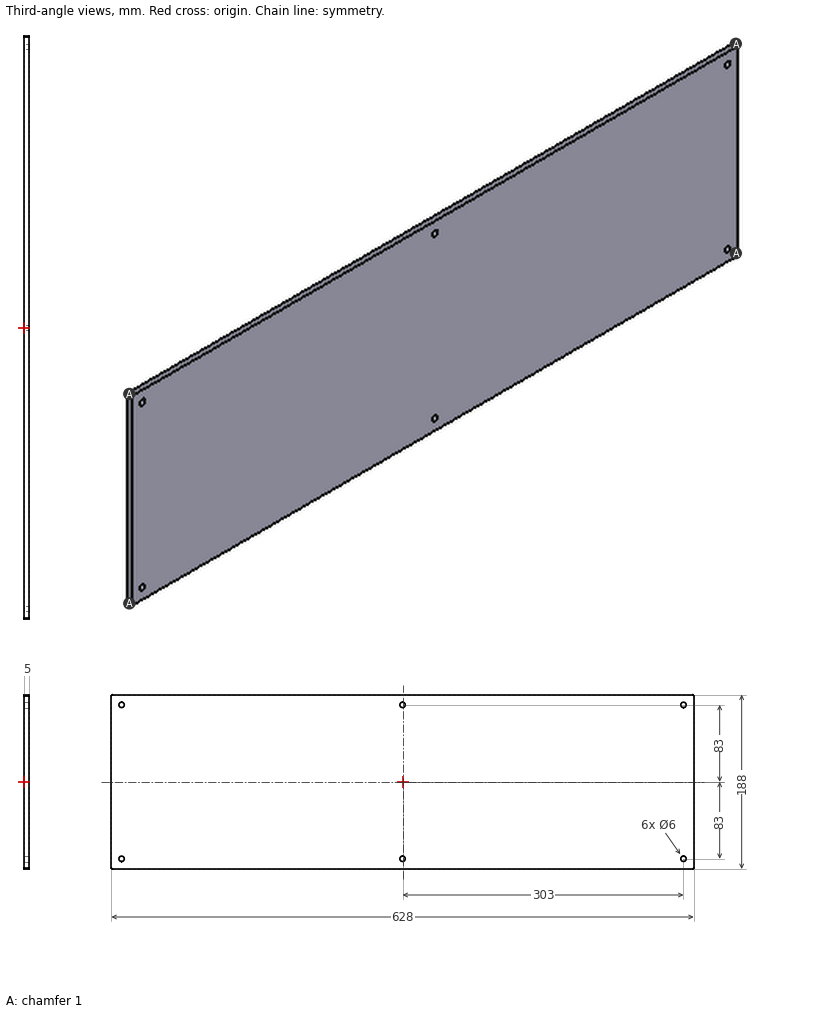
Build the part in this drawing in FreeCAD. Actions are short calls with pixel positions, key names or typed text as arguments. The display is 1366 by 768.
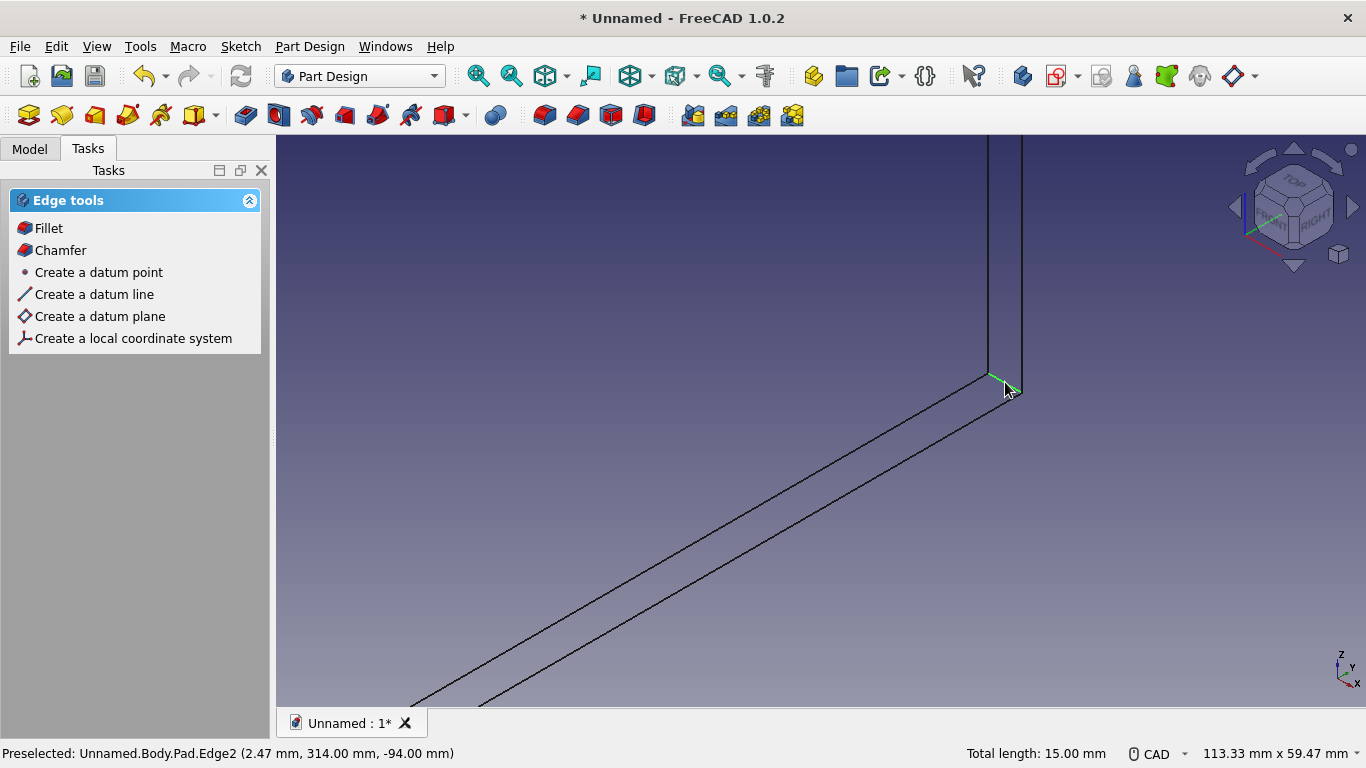
key(v)
key(f)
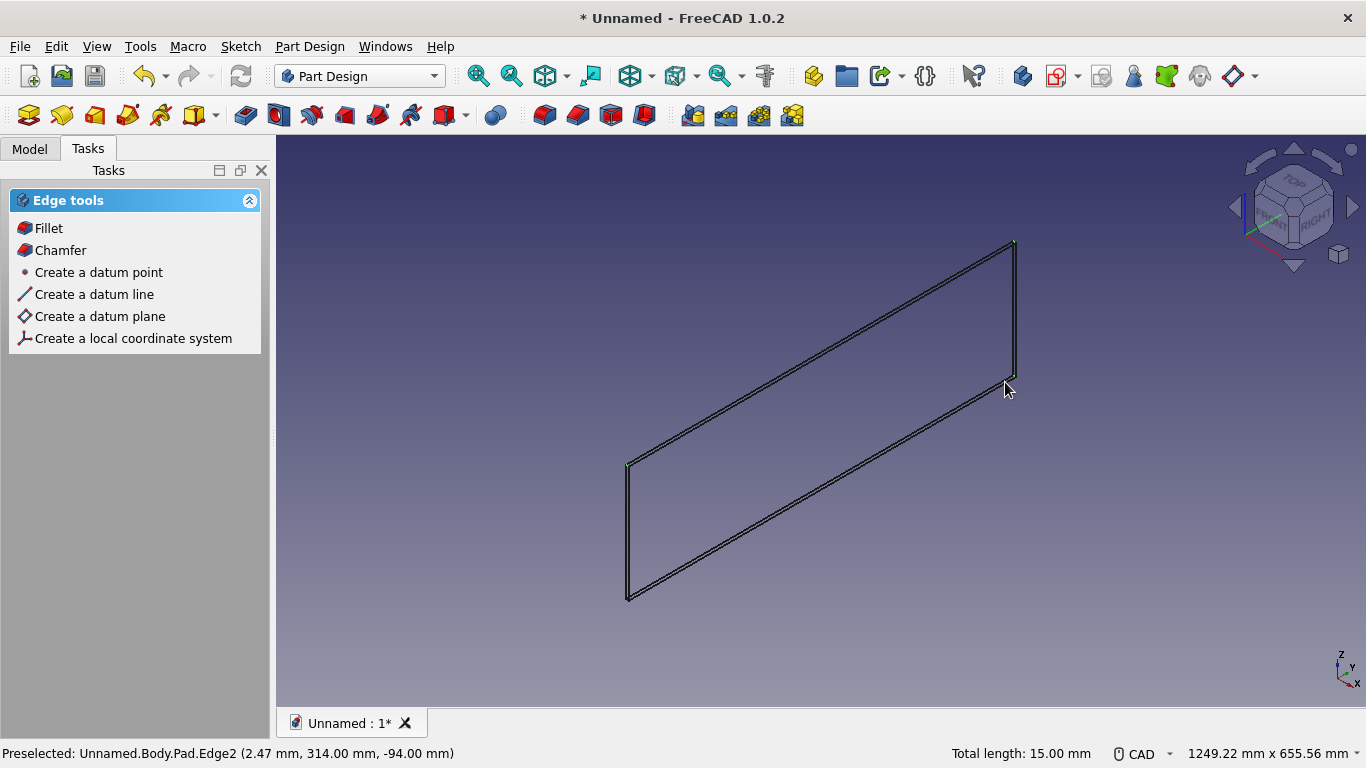
key(2)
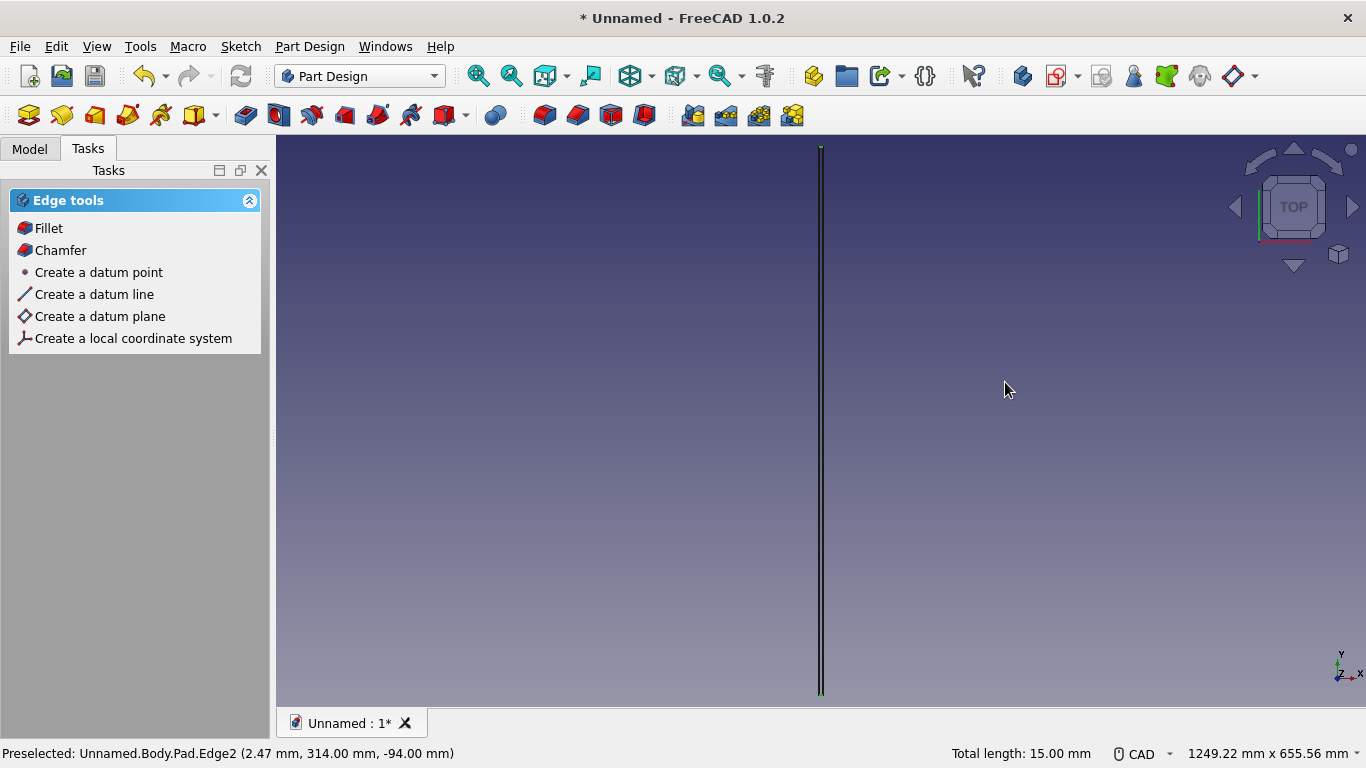
key(1)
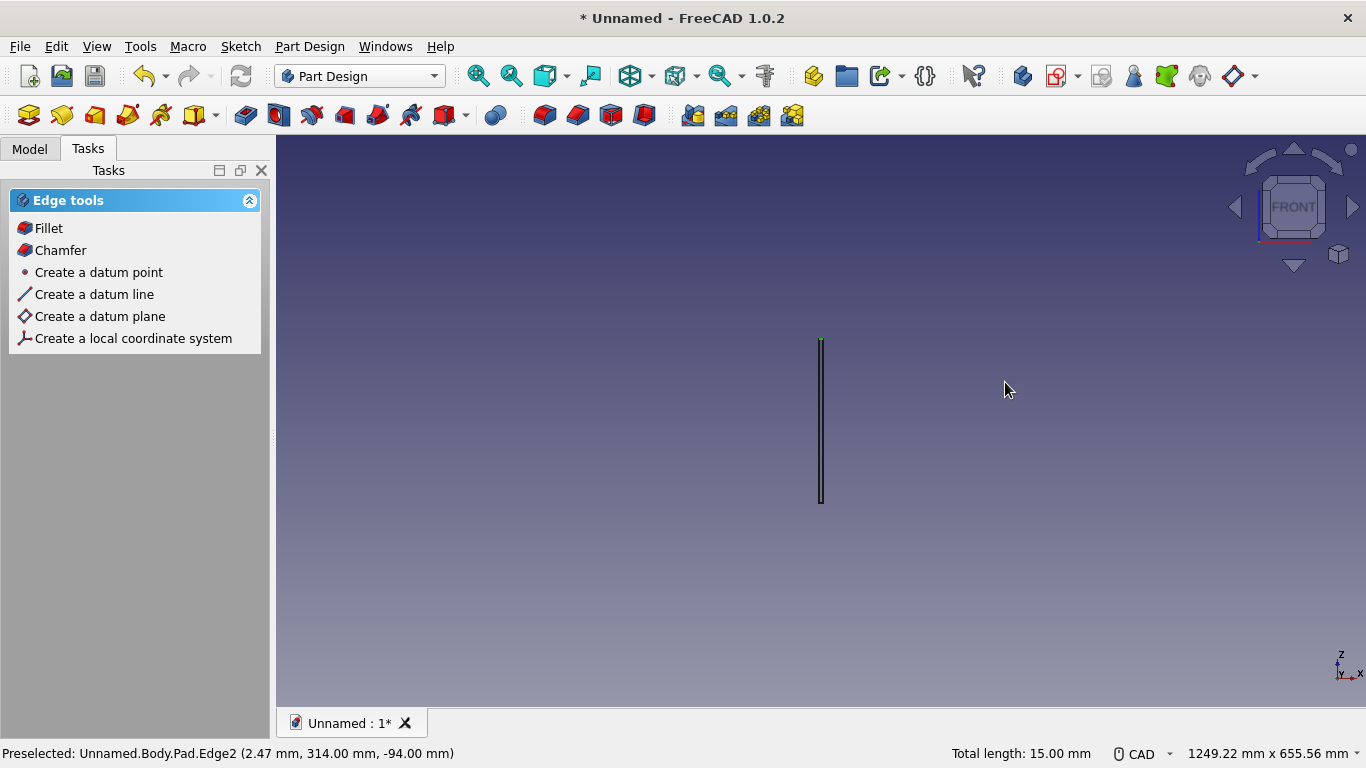
key(v)
key(f)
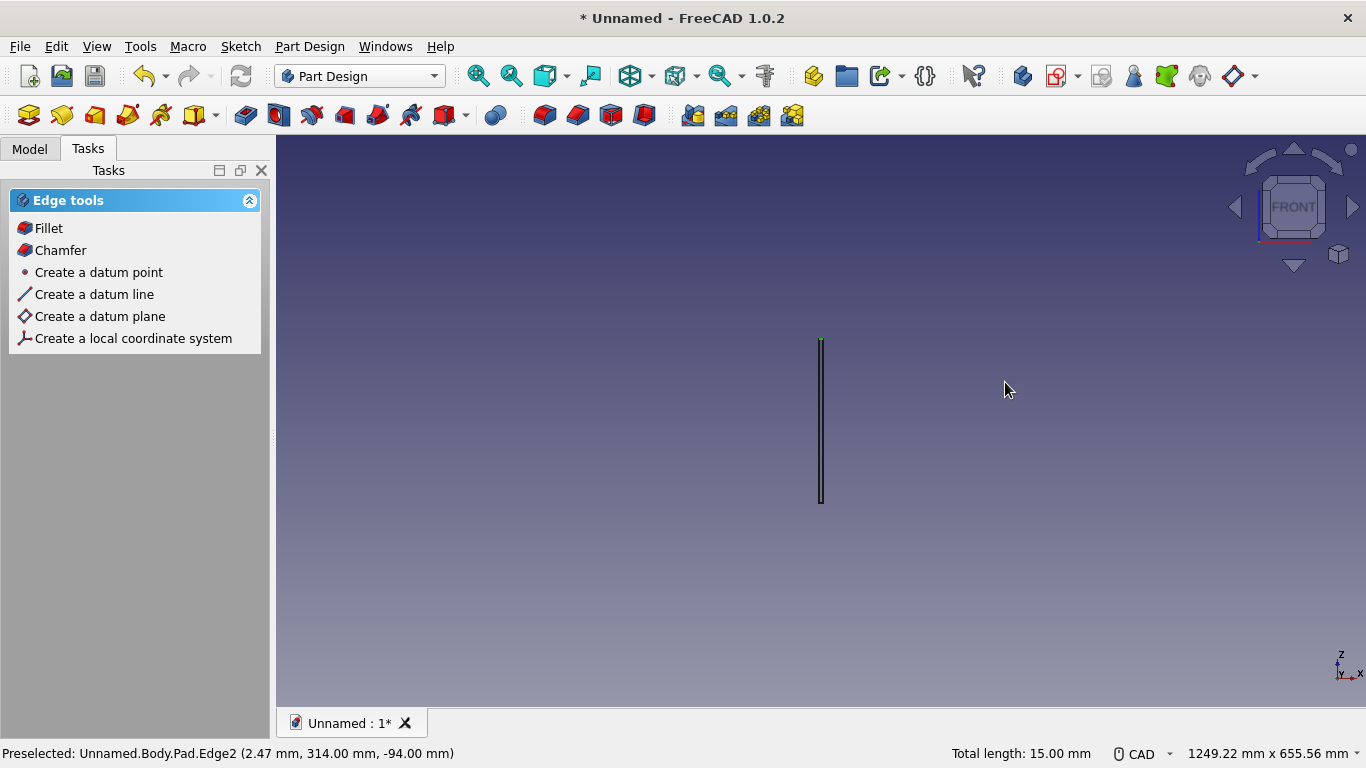
click(821, 502, ctrl)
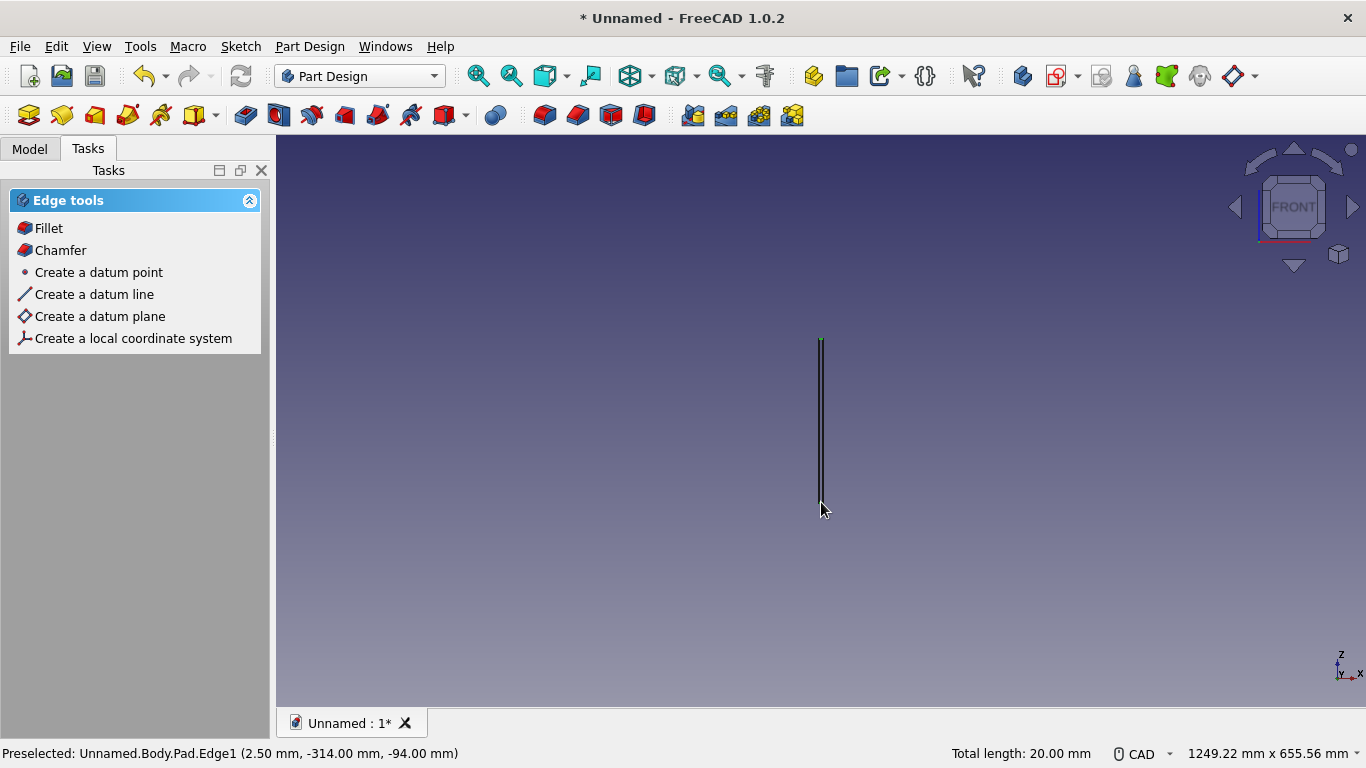
key(v)
key(1)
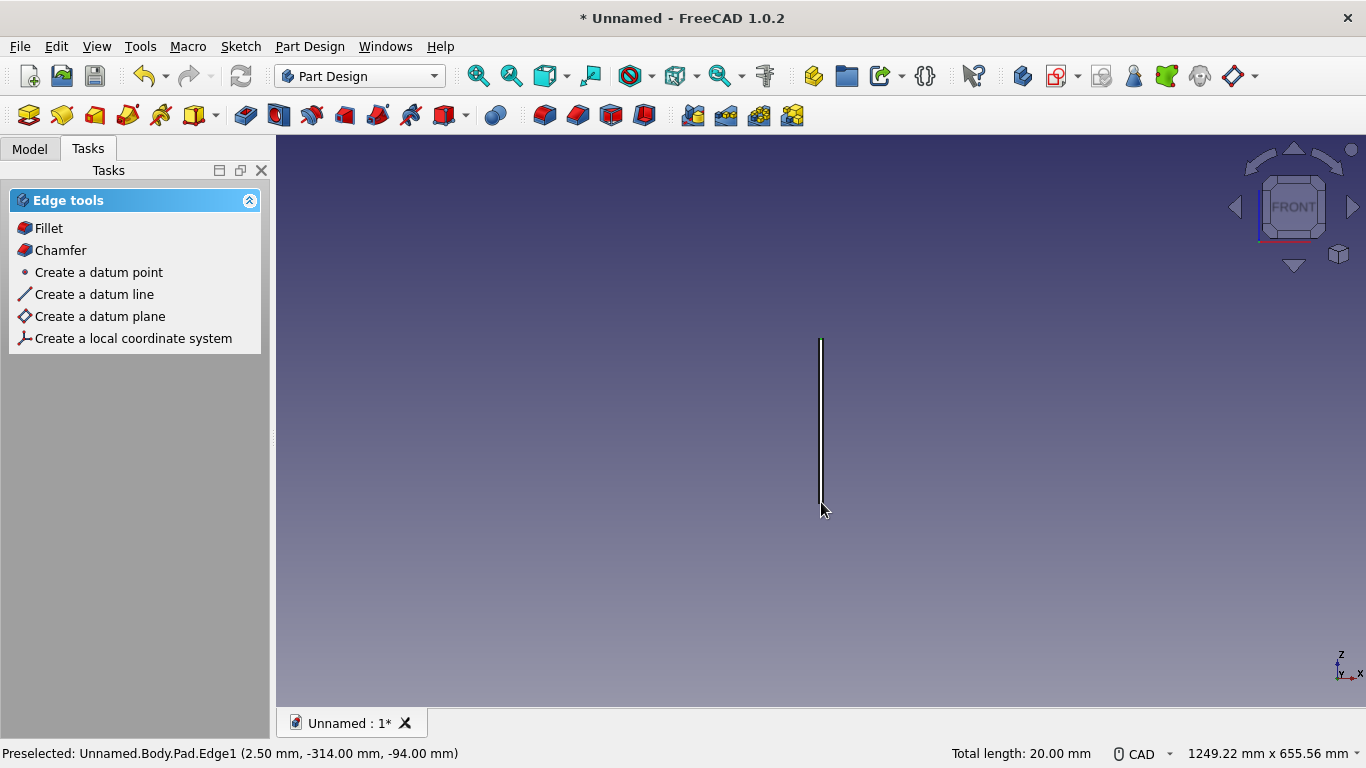
click(578, 116)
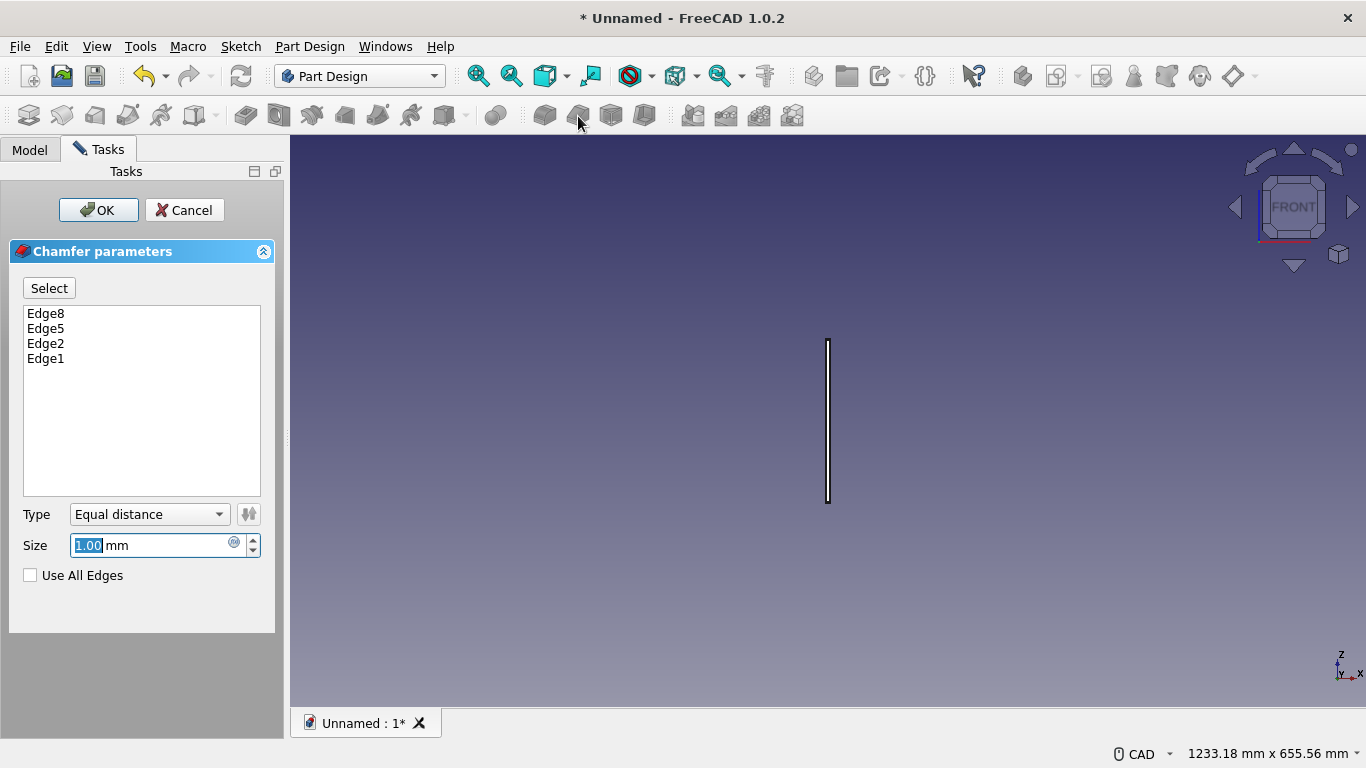
text(1)
key(Tab)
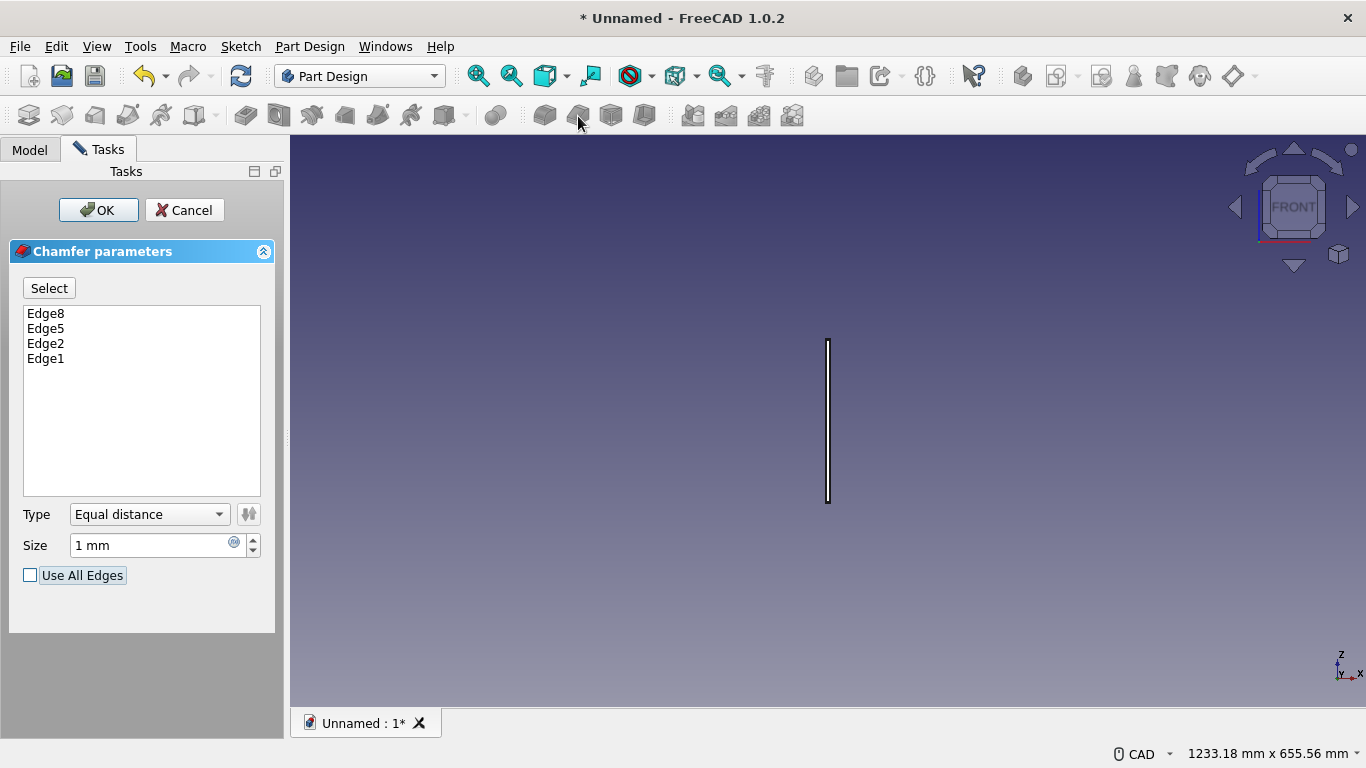
click(99, 210)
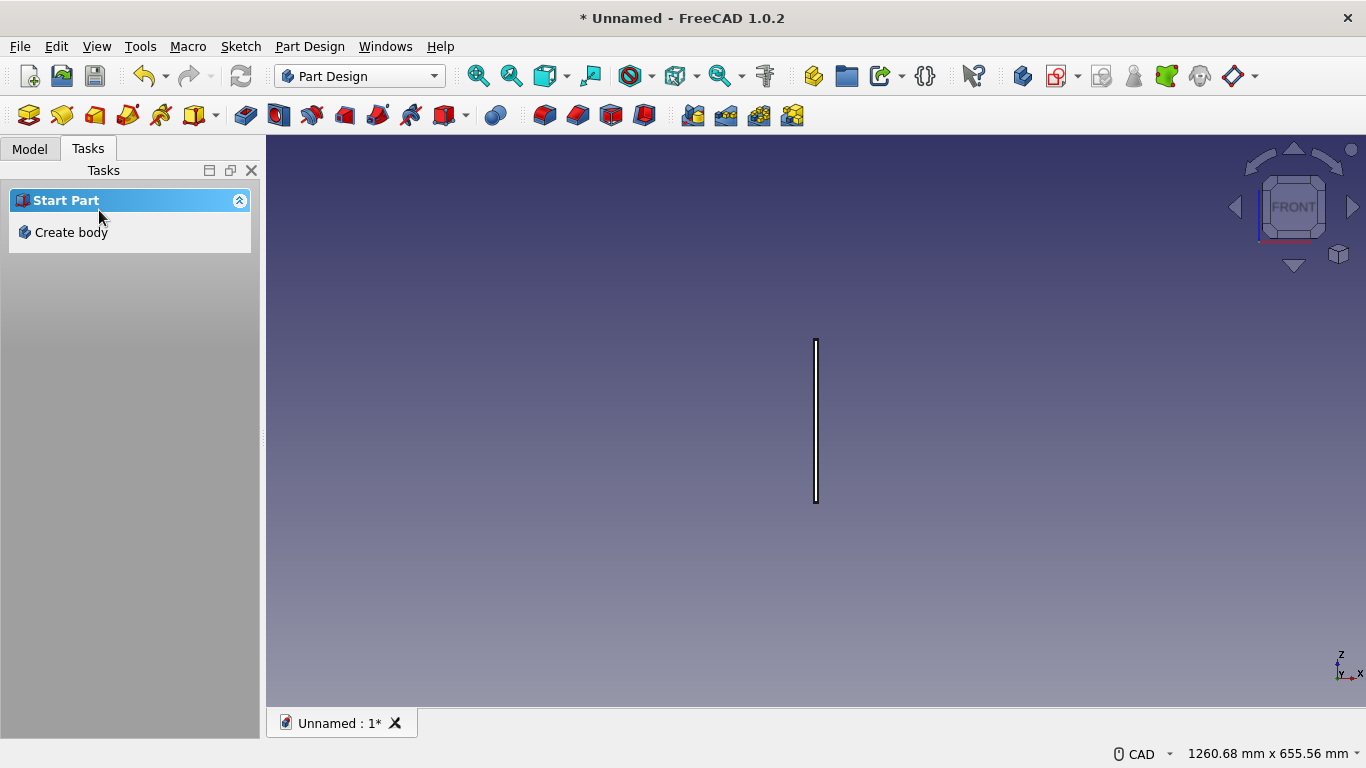
key(v)
key(f)